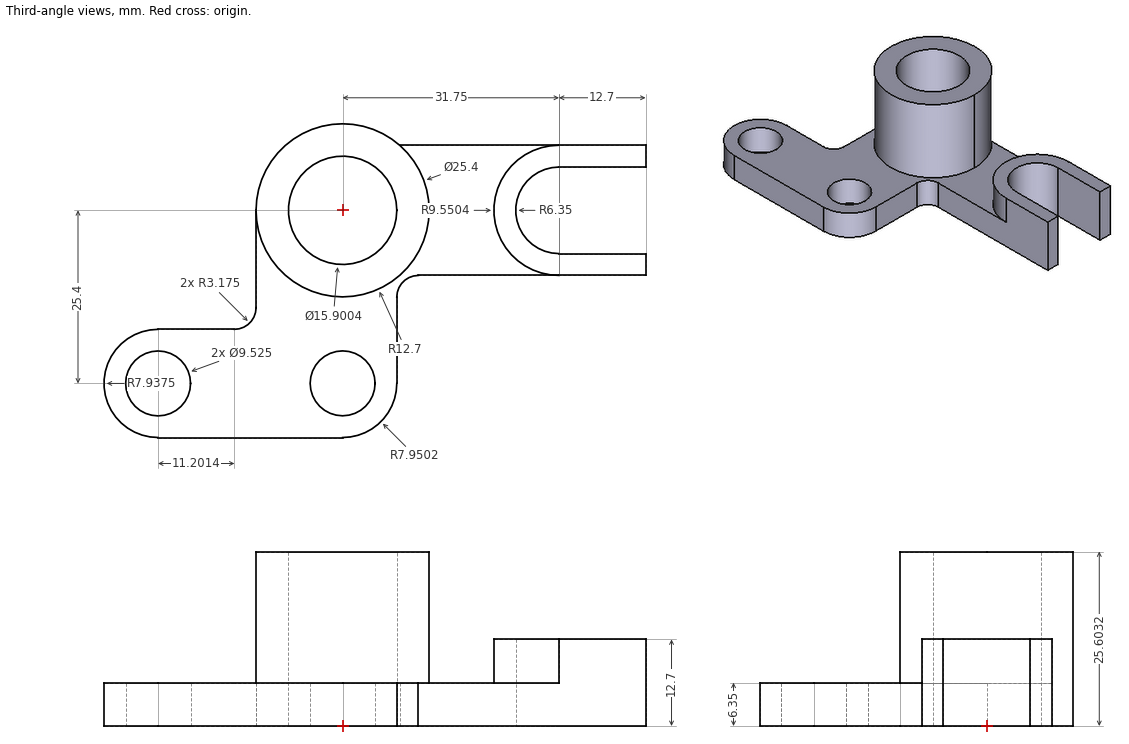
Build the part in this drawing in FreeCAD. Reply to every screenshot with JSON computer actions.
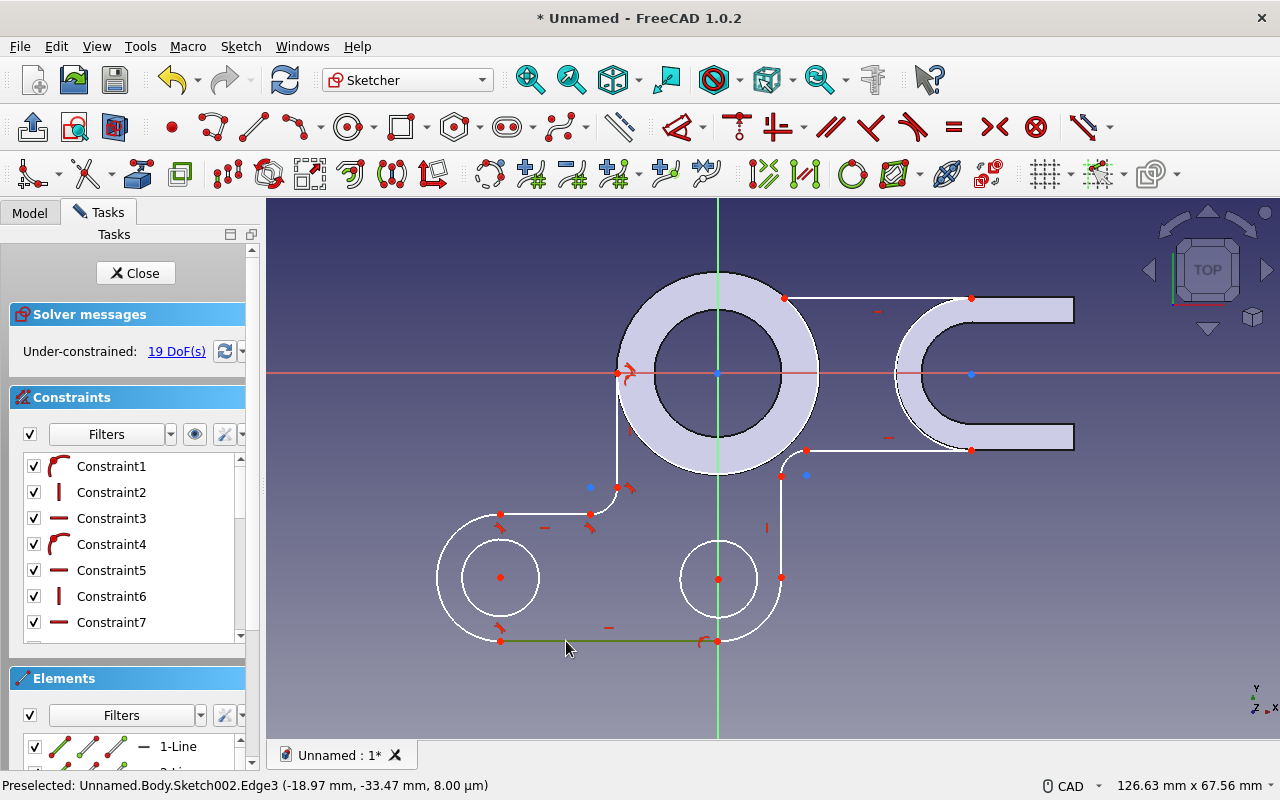
{"action": "left_click", "coordinate": [747, 635]}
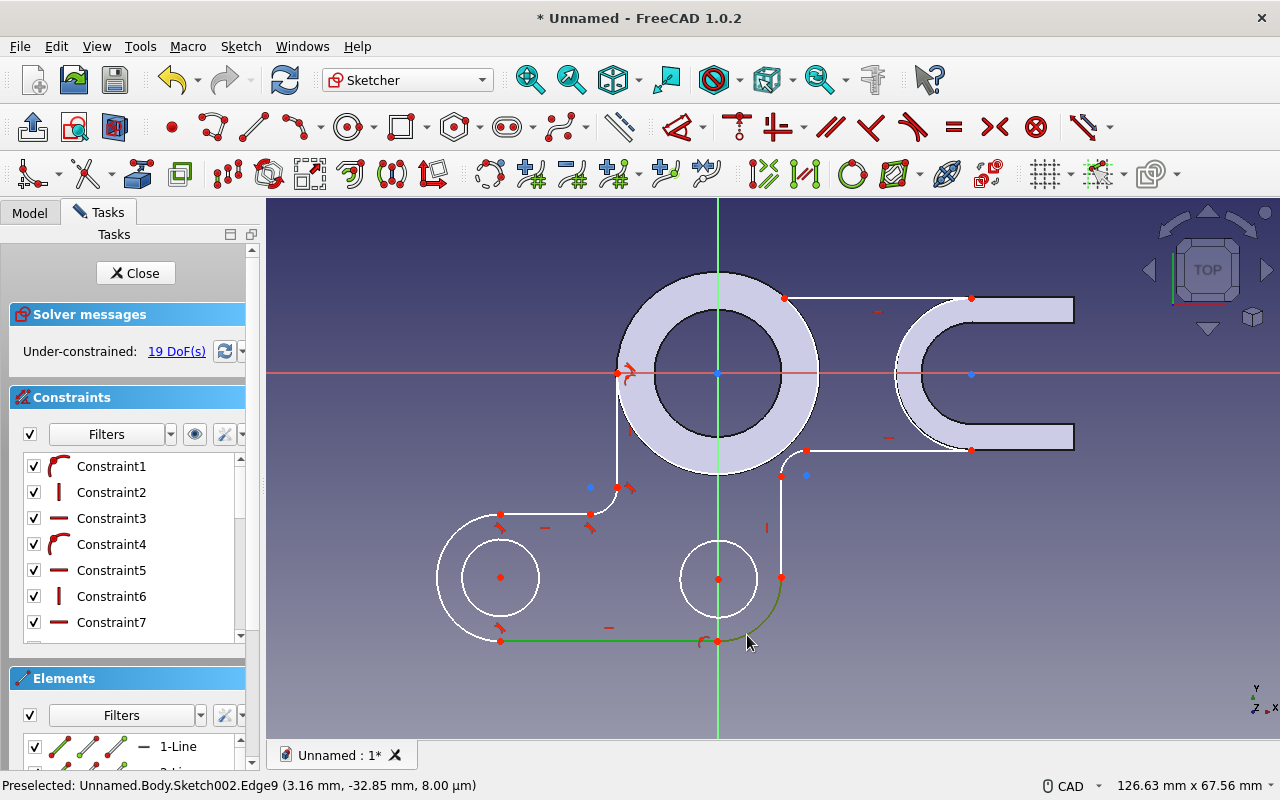
{"action": "key", "text": "t"}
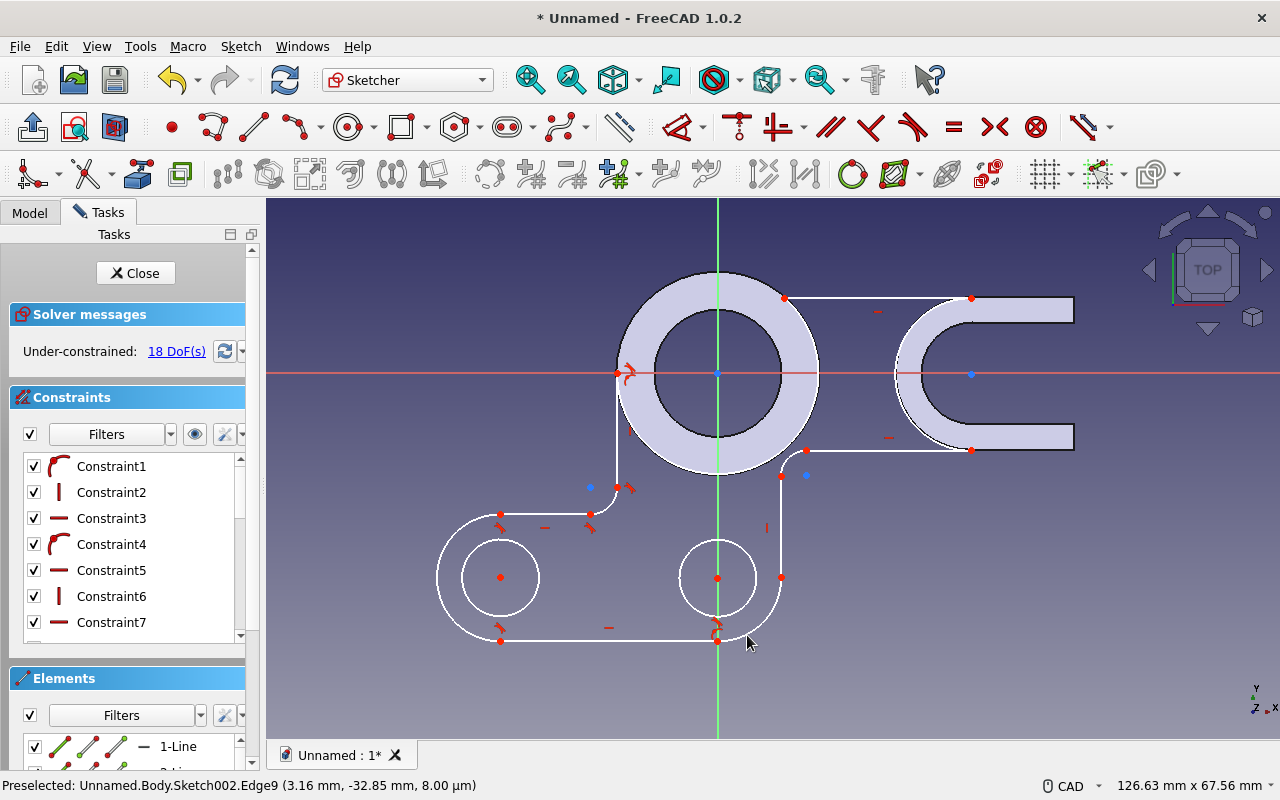
{"action": "left_click", "coordinate": [781, 547]}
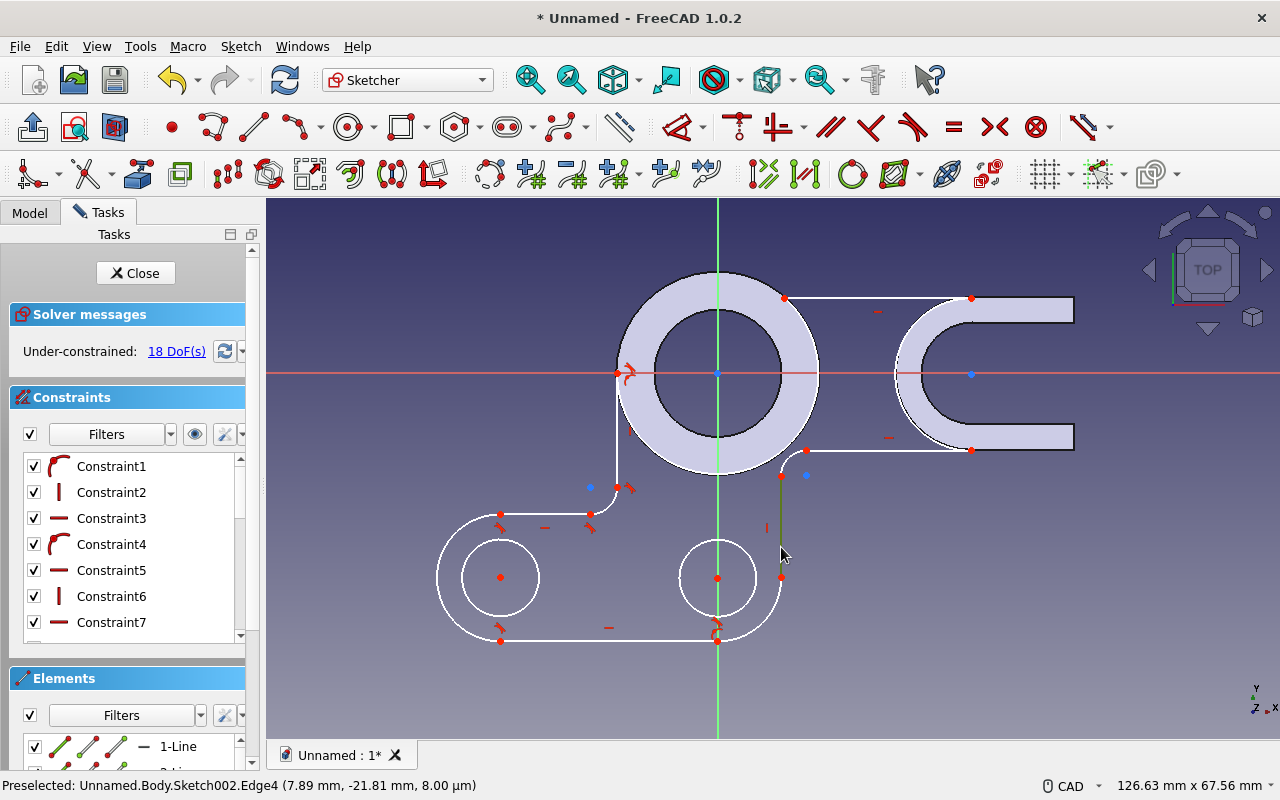
{"action": "left_click", "coordinate": [747, 634]}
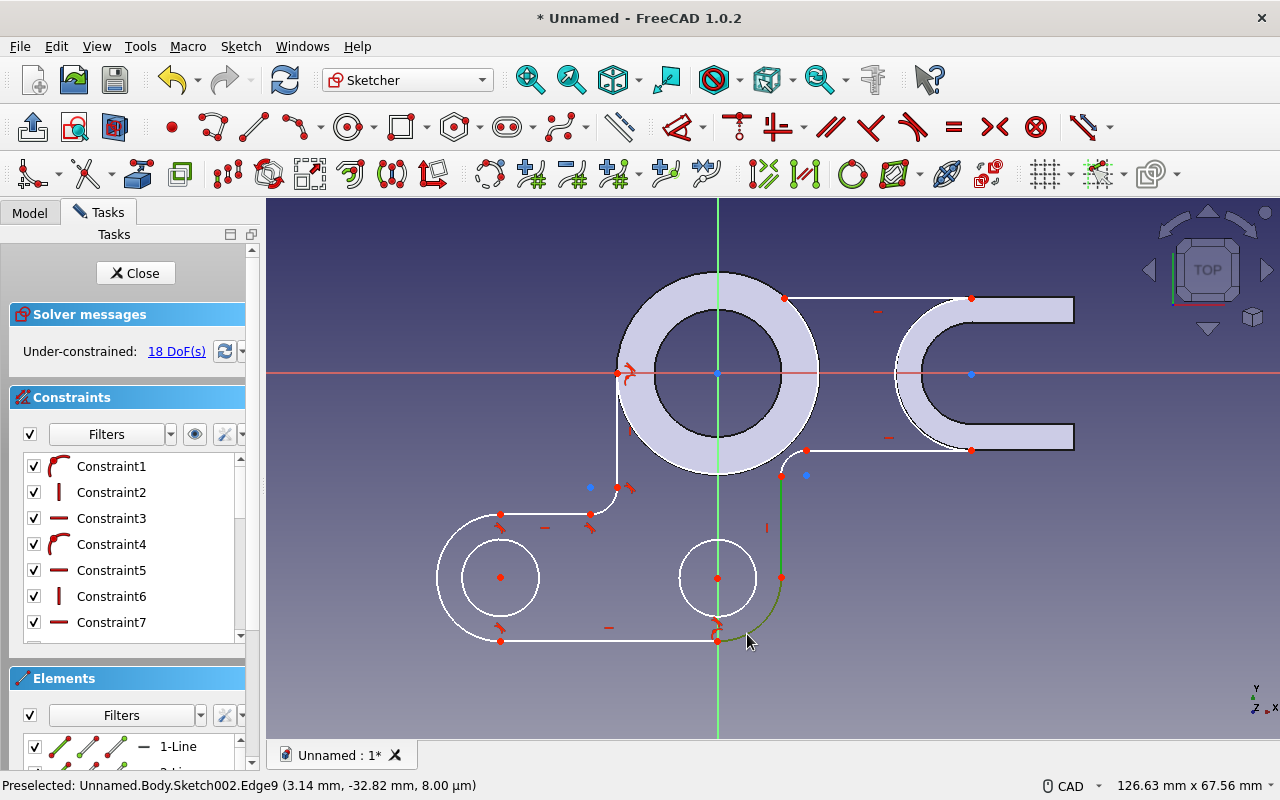
{"action": "key", "text": "t"}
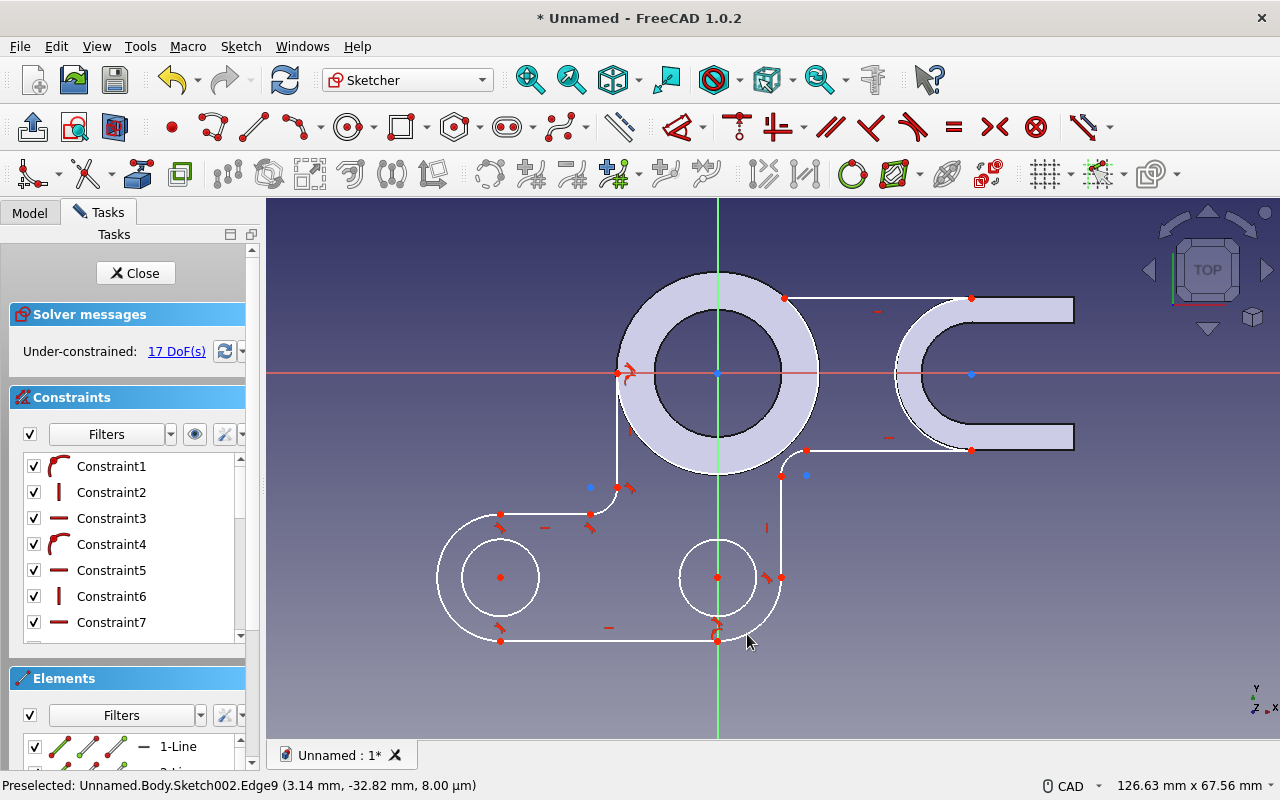
{"action": "left_click", "coordinate": [781, 547]}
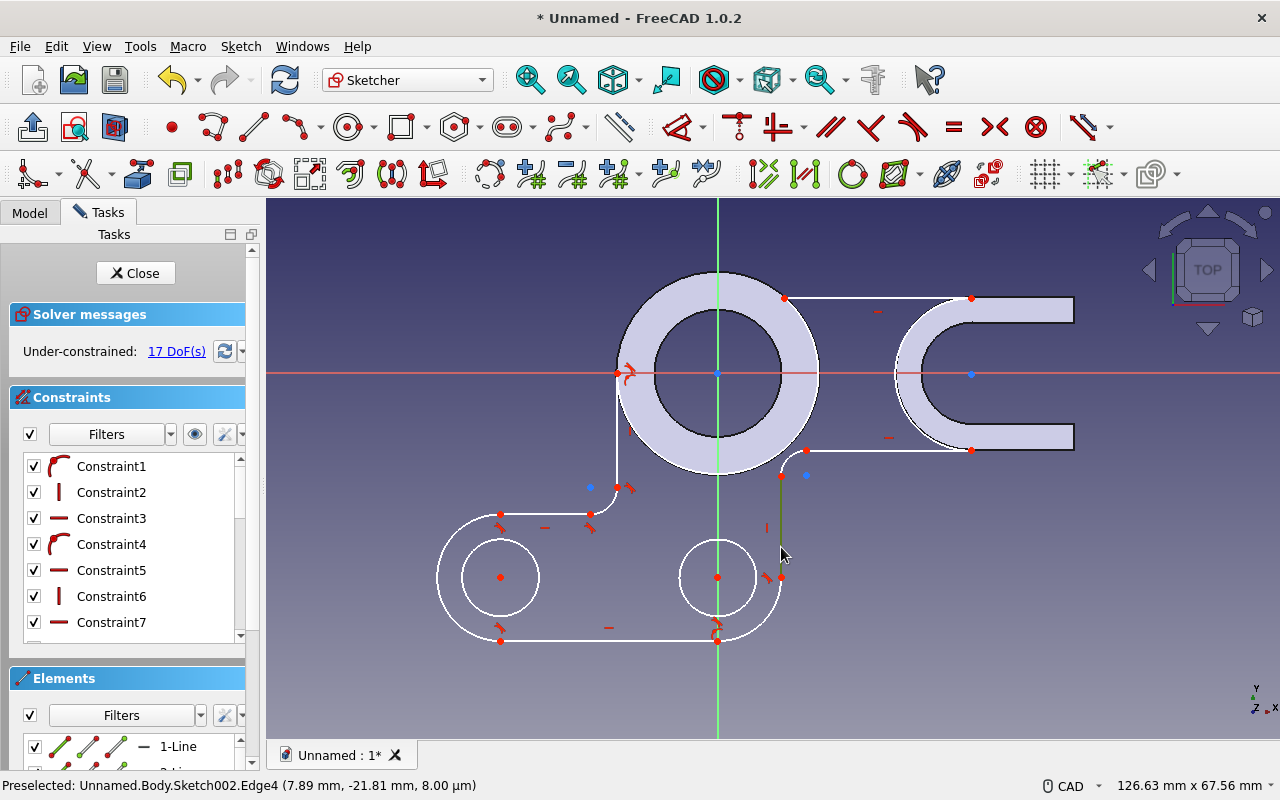
{"action": "scroll", "coordinate": [795, 453], "scroll_direction": "up", "scroll_amount": 2}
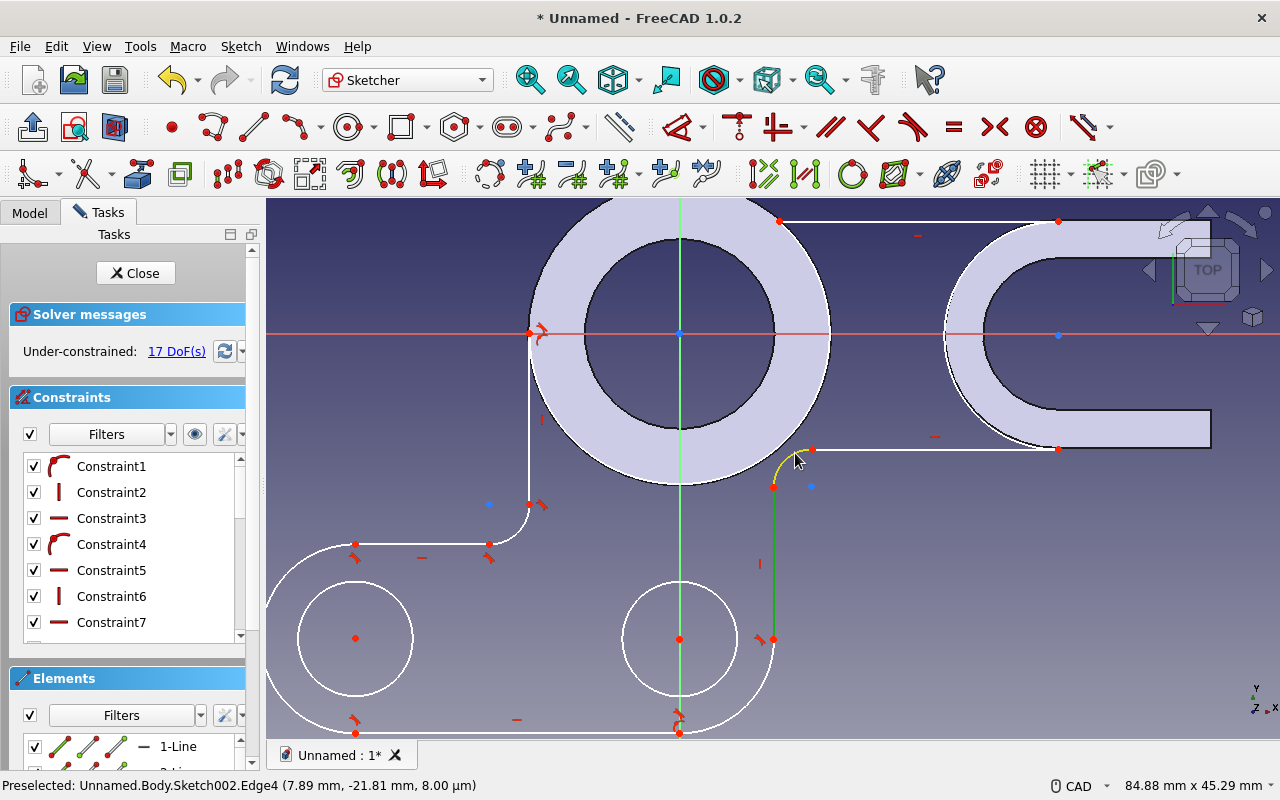
{"action": "left_click", "coordinate": [795, 453]}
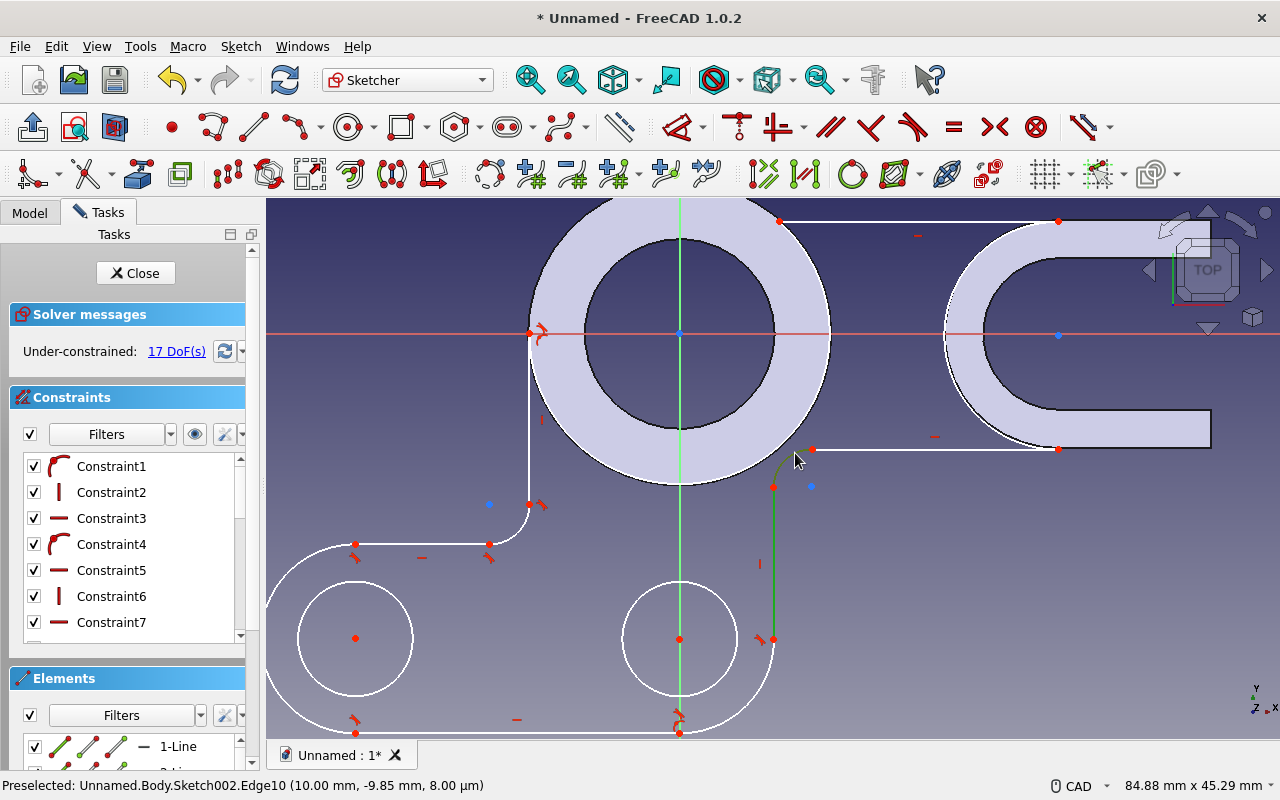
{"action": "left_click", "coordinate": [913, 128]}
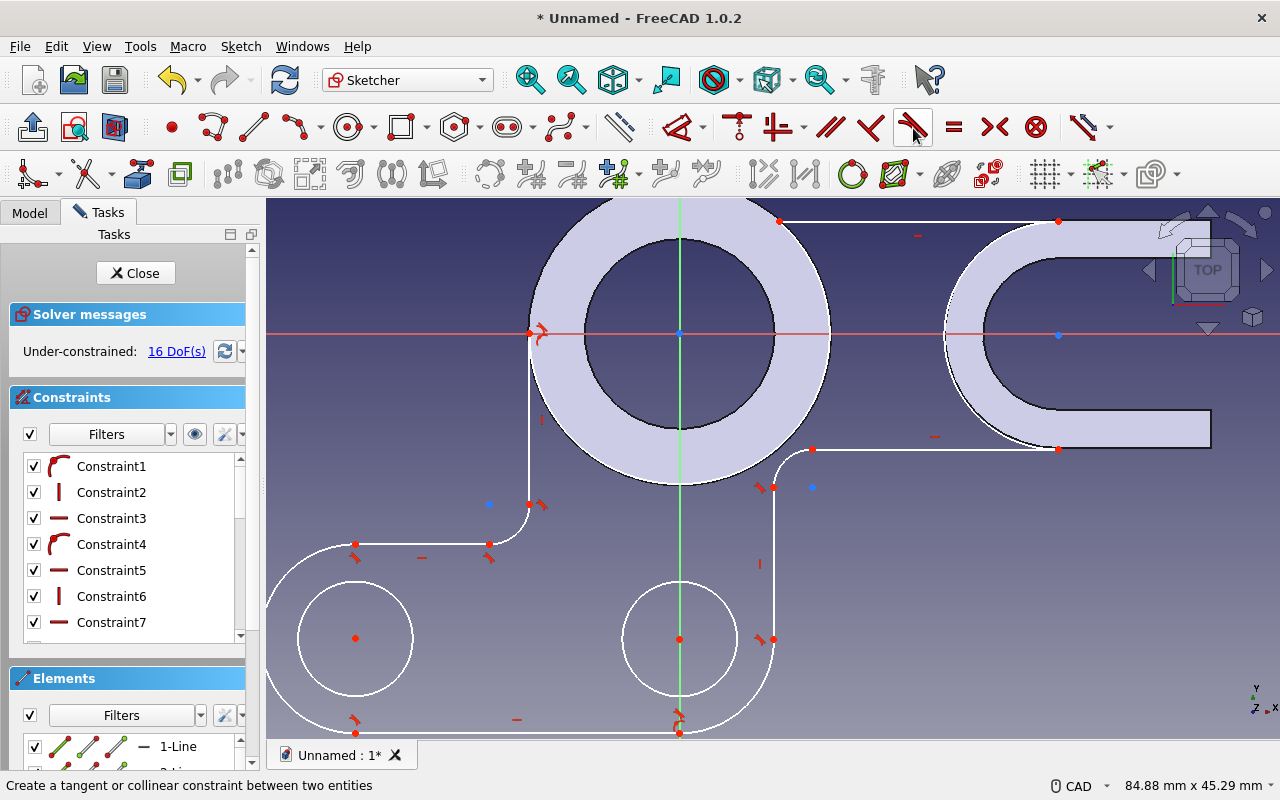
{"action": "left_click", "coordinate": [886, 450]}